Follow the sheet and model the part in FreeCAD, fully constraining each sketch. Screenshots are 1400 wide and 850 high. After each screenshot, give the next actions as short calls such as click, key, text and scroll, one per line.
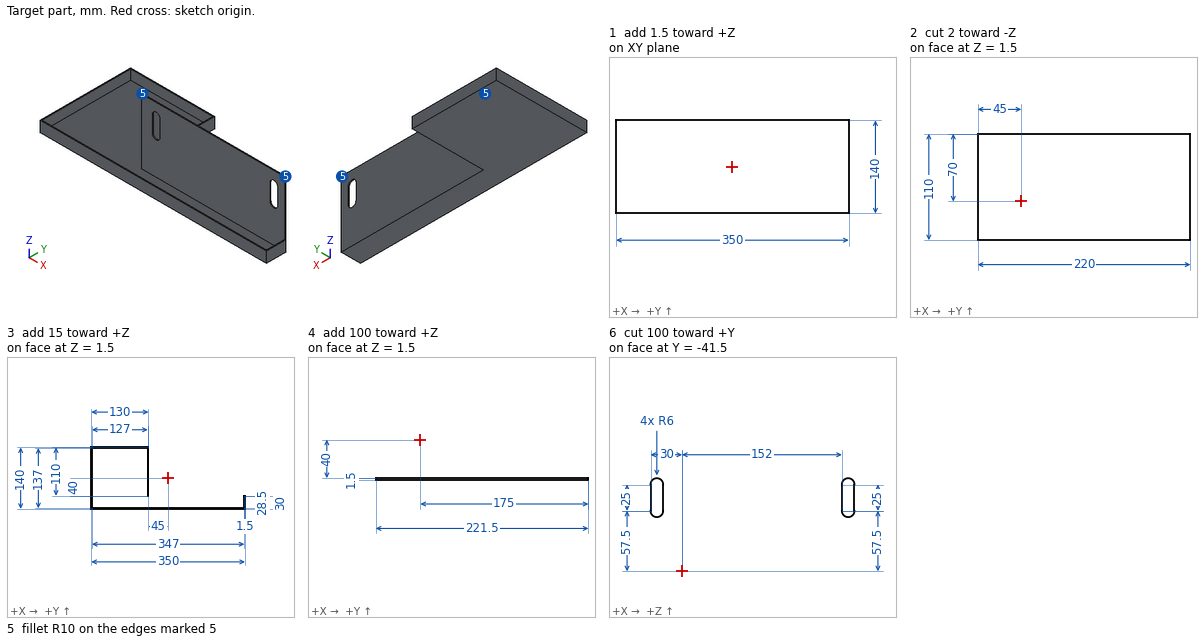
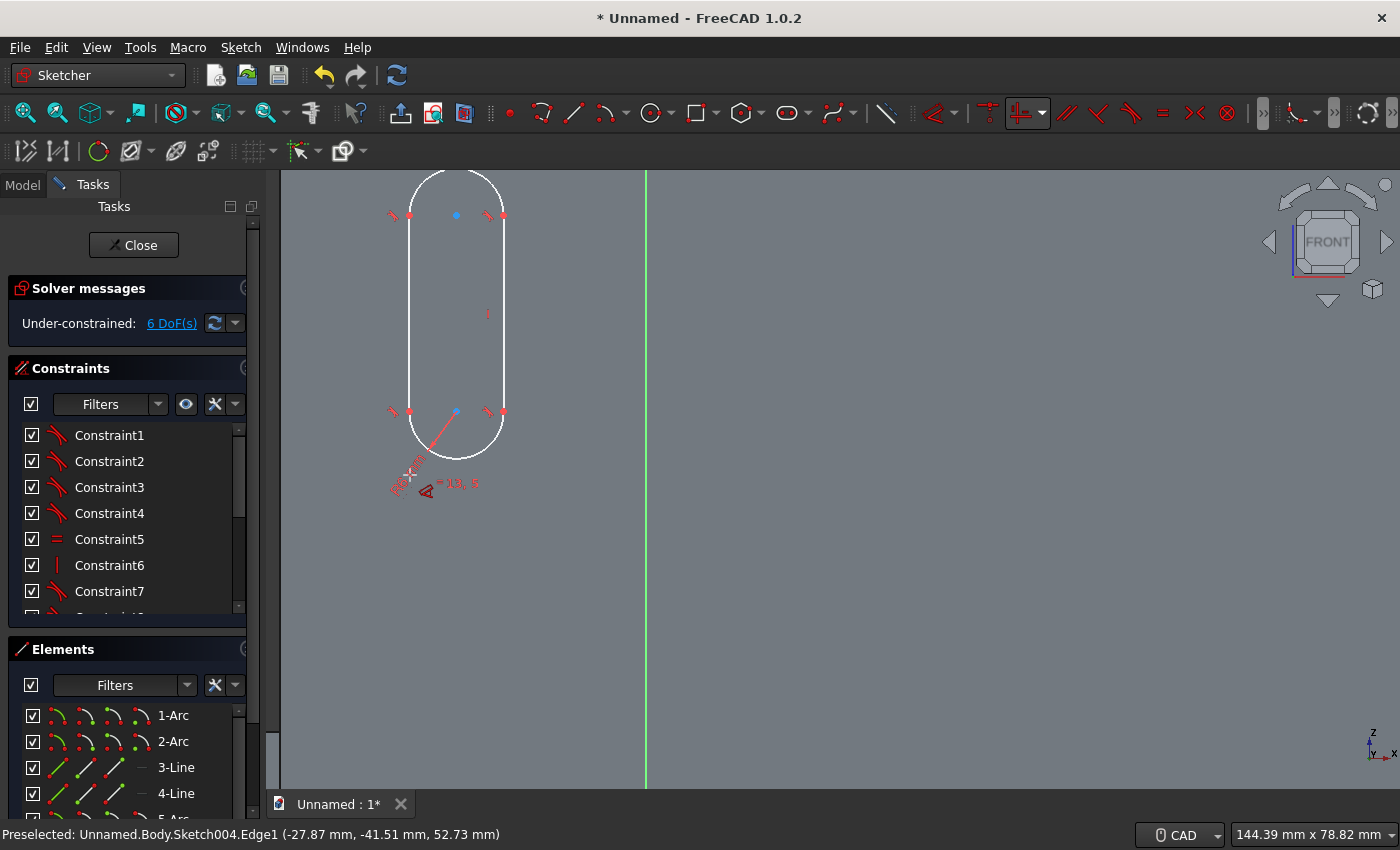
click(409, 353)
click(375, 314)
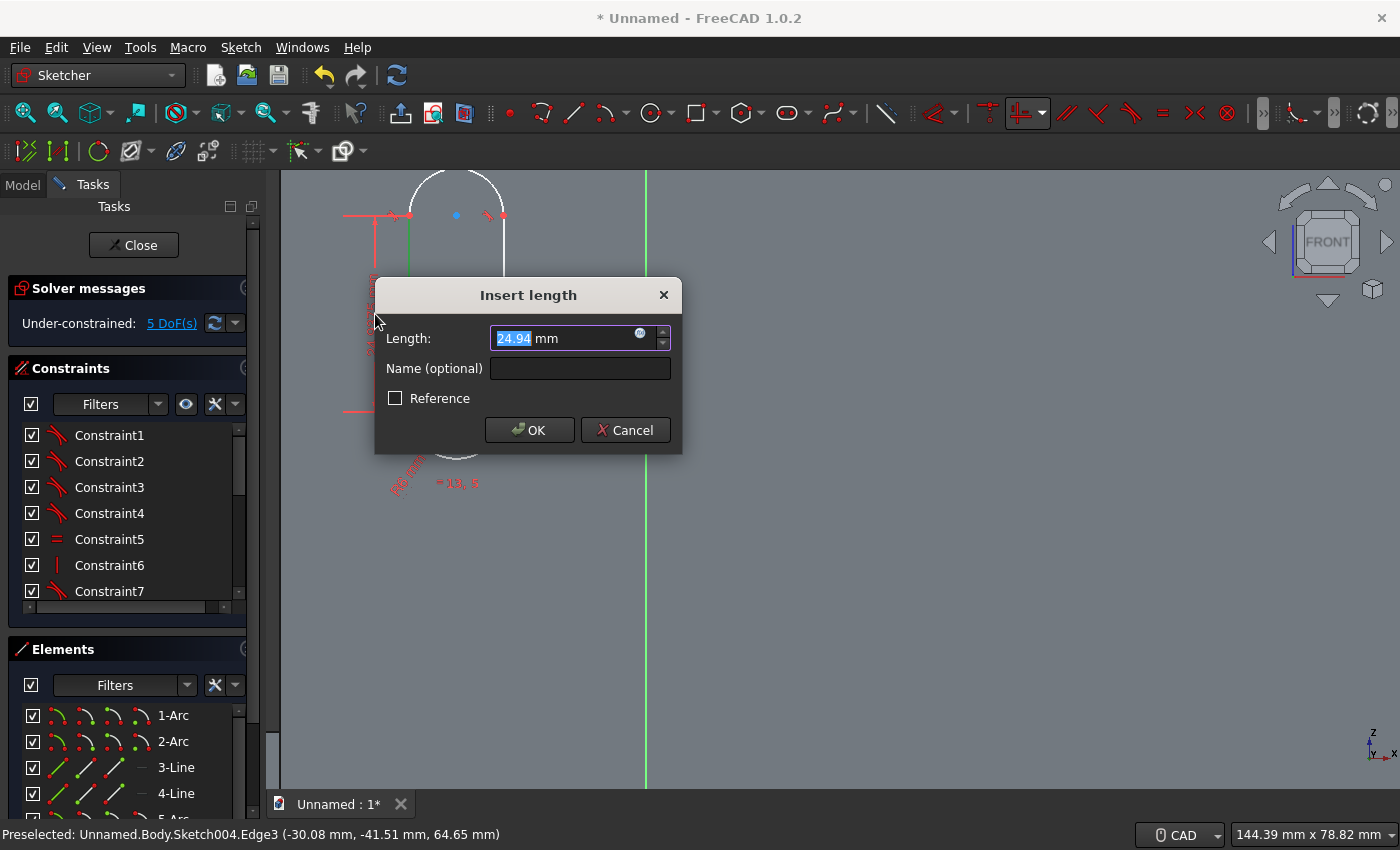
text(25)
key(Return)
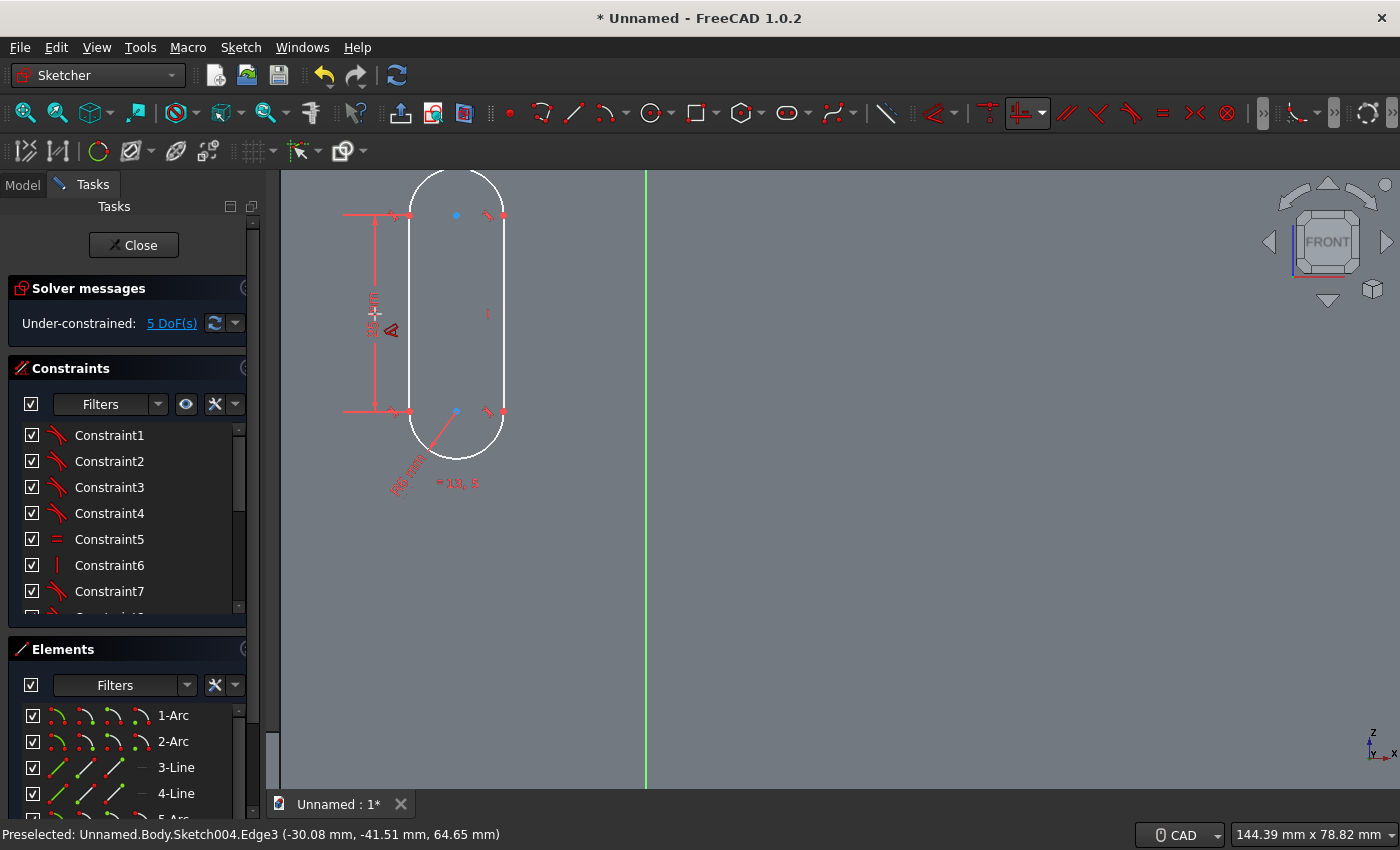
scroll(432, 451, down, 4)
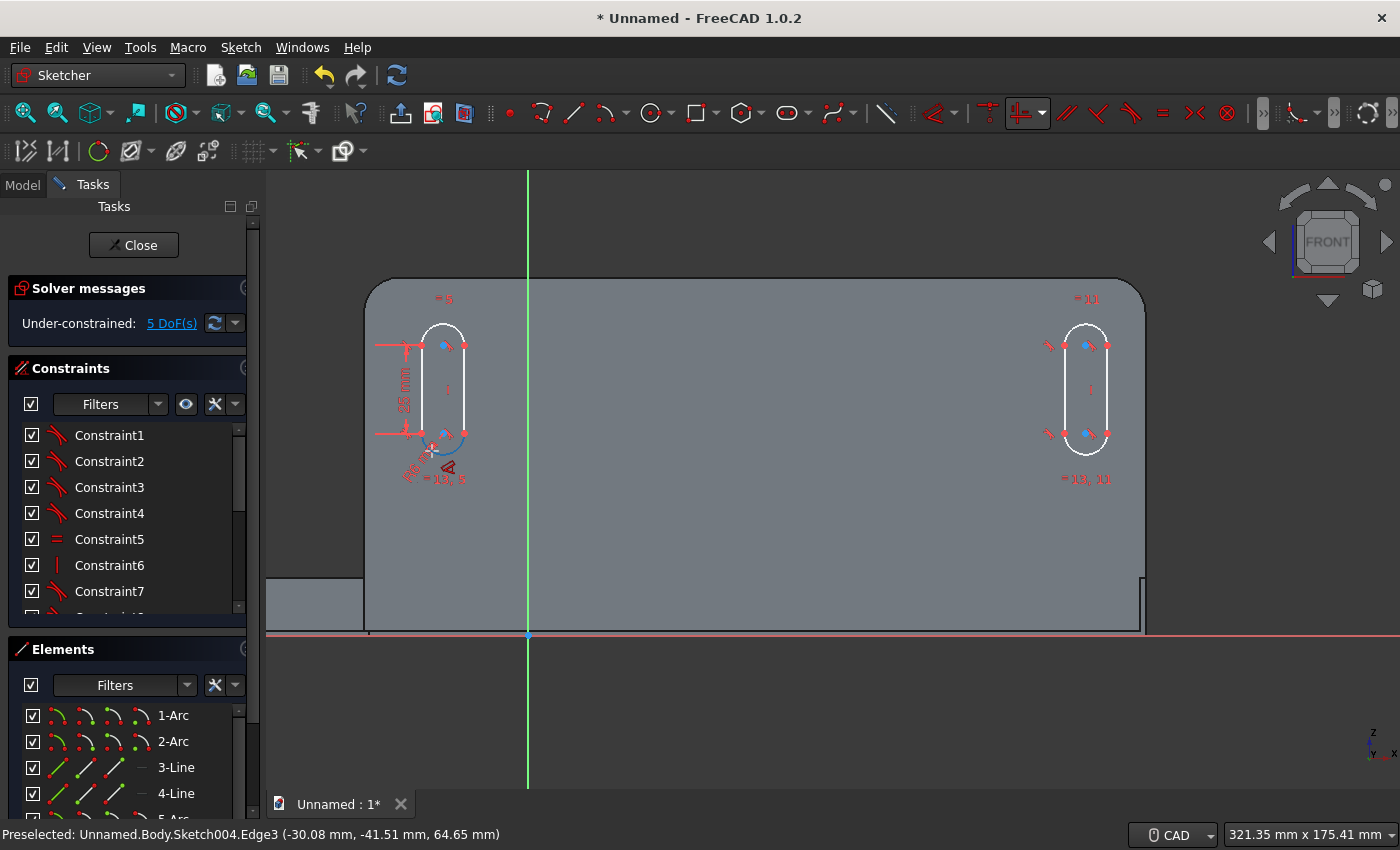
click(1065, 407)
click(1031, 390)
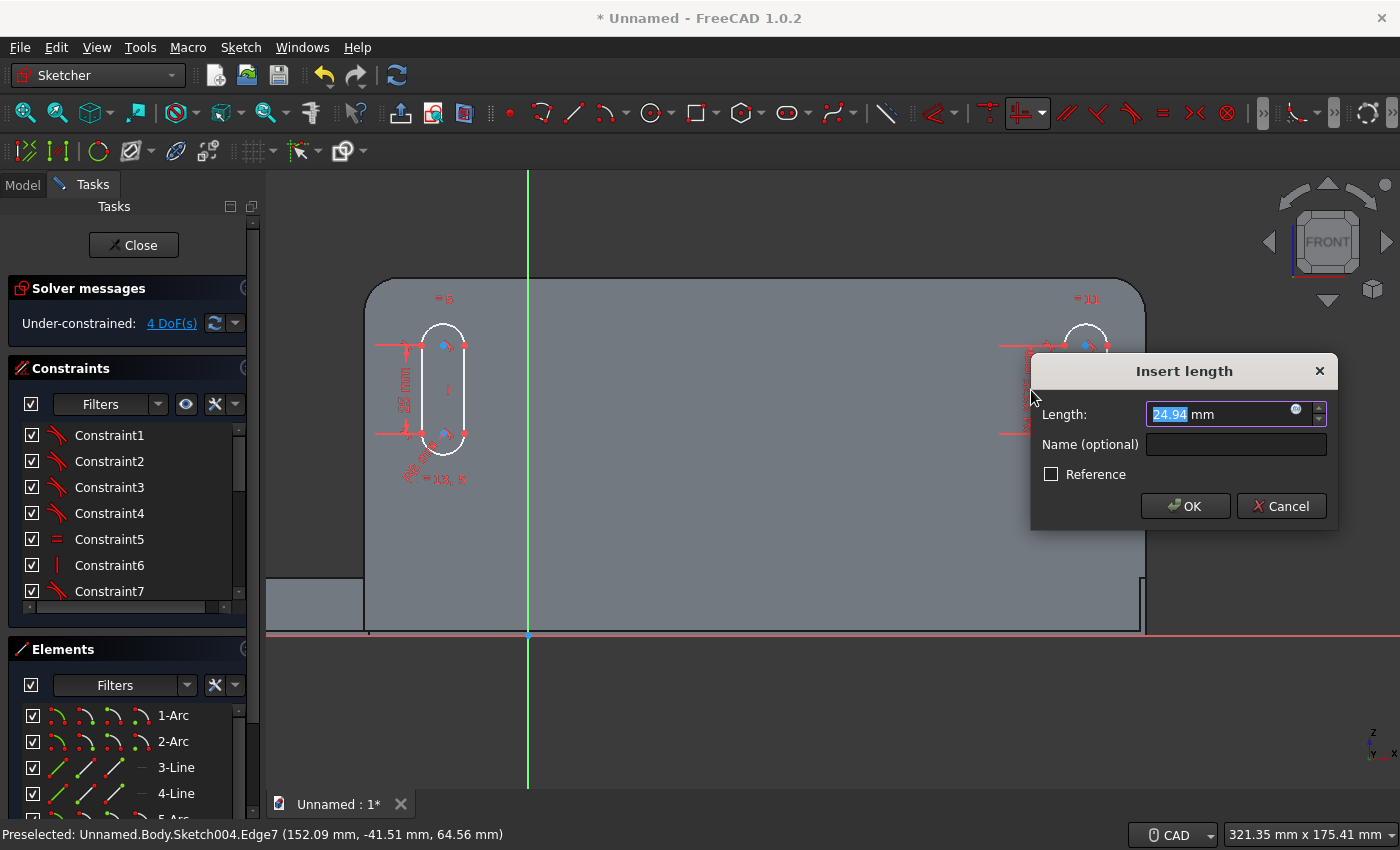
text(25)
key(Return)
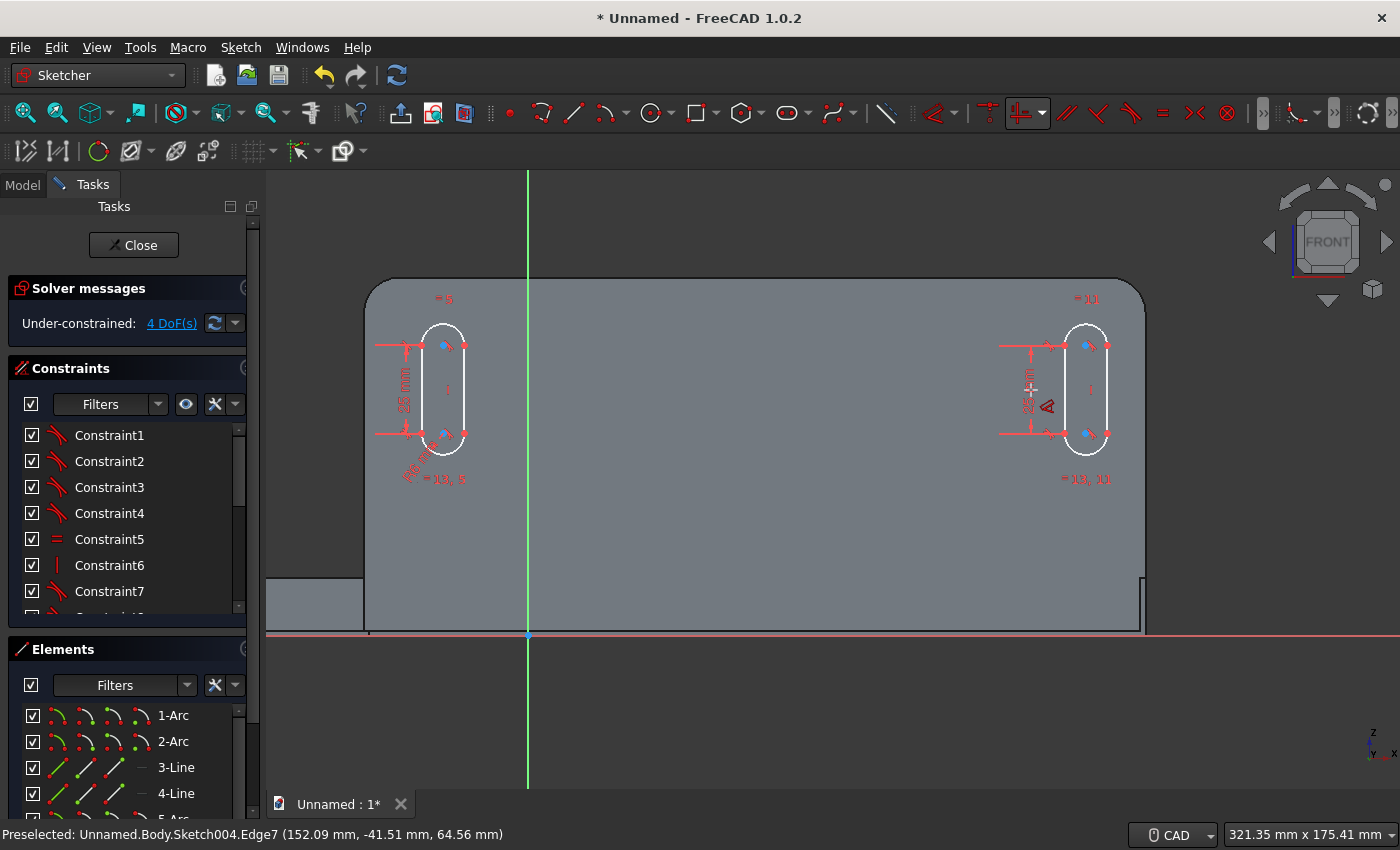
click(422, 434)
click(475, 670)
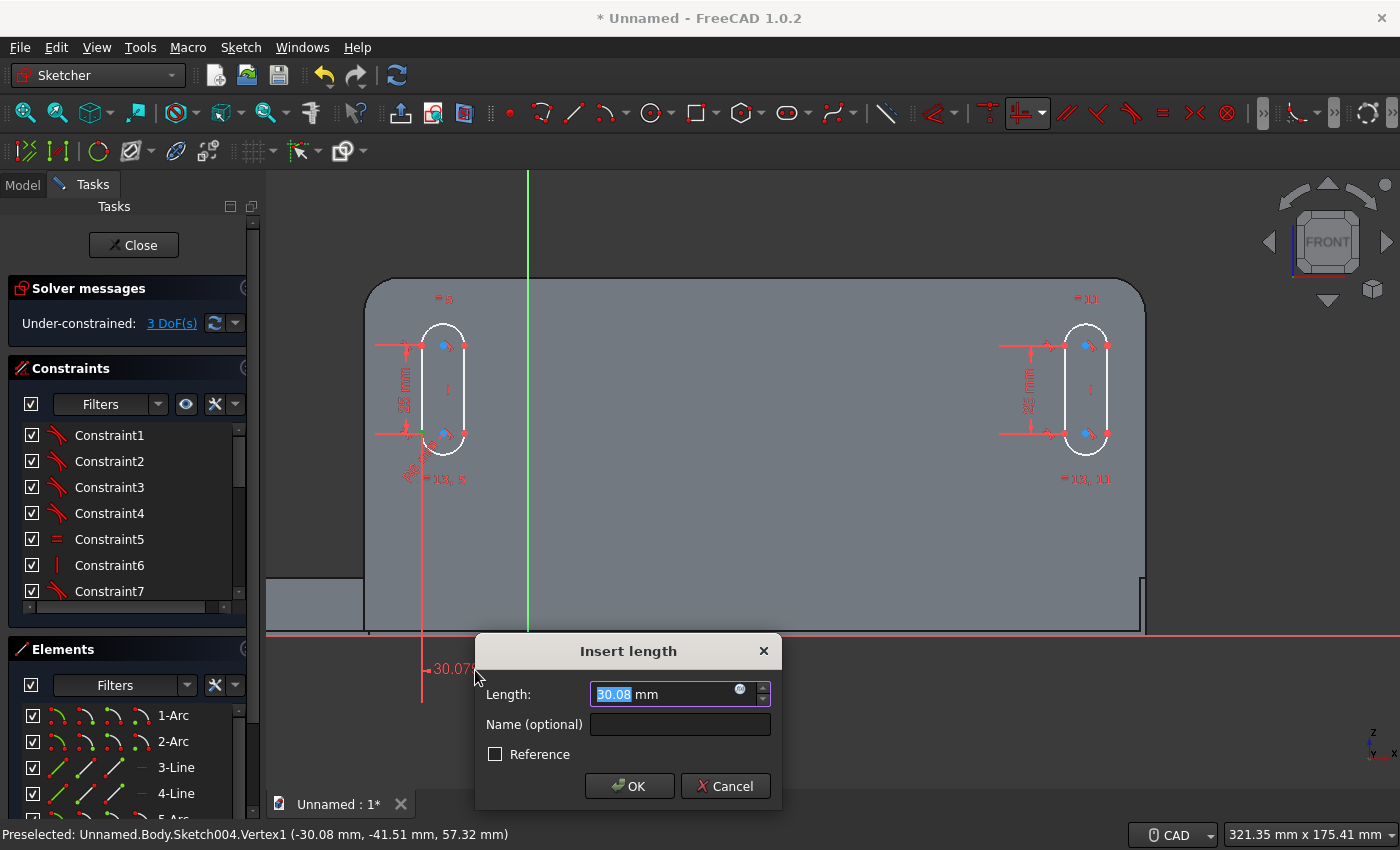
text(30)
key(Return)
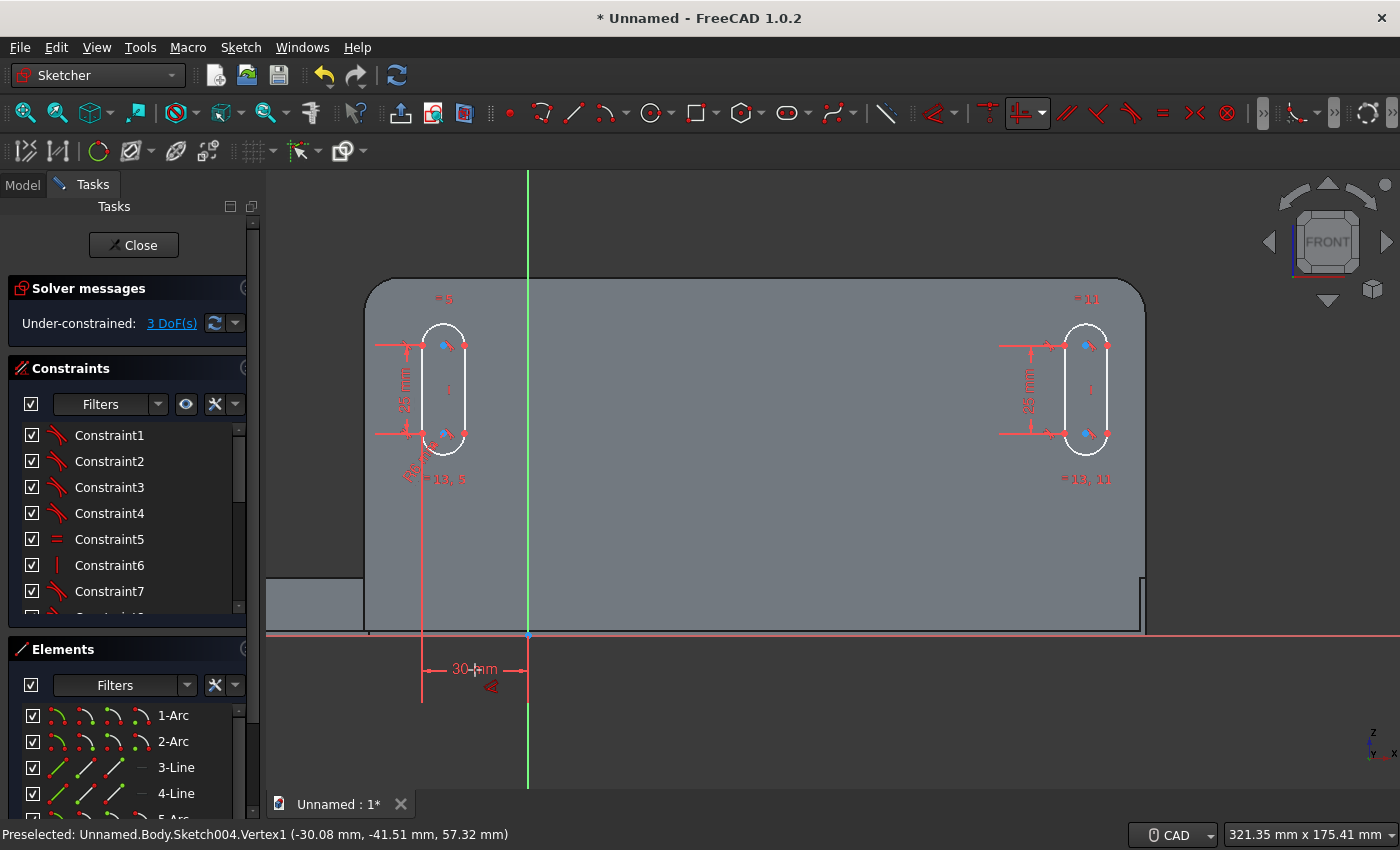
click(1065, 434)
click(796, 670)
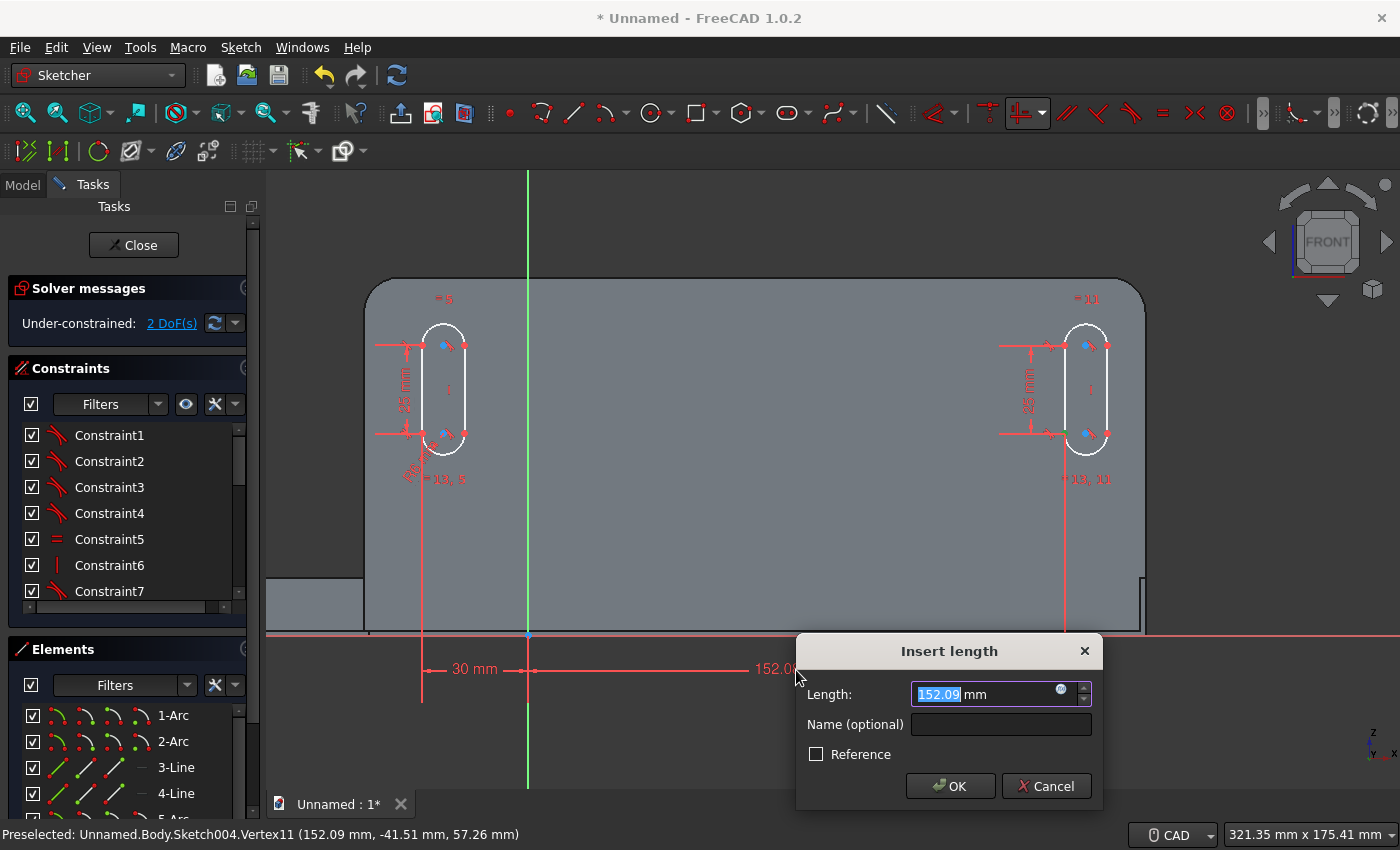
text(152)
key(Return)